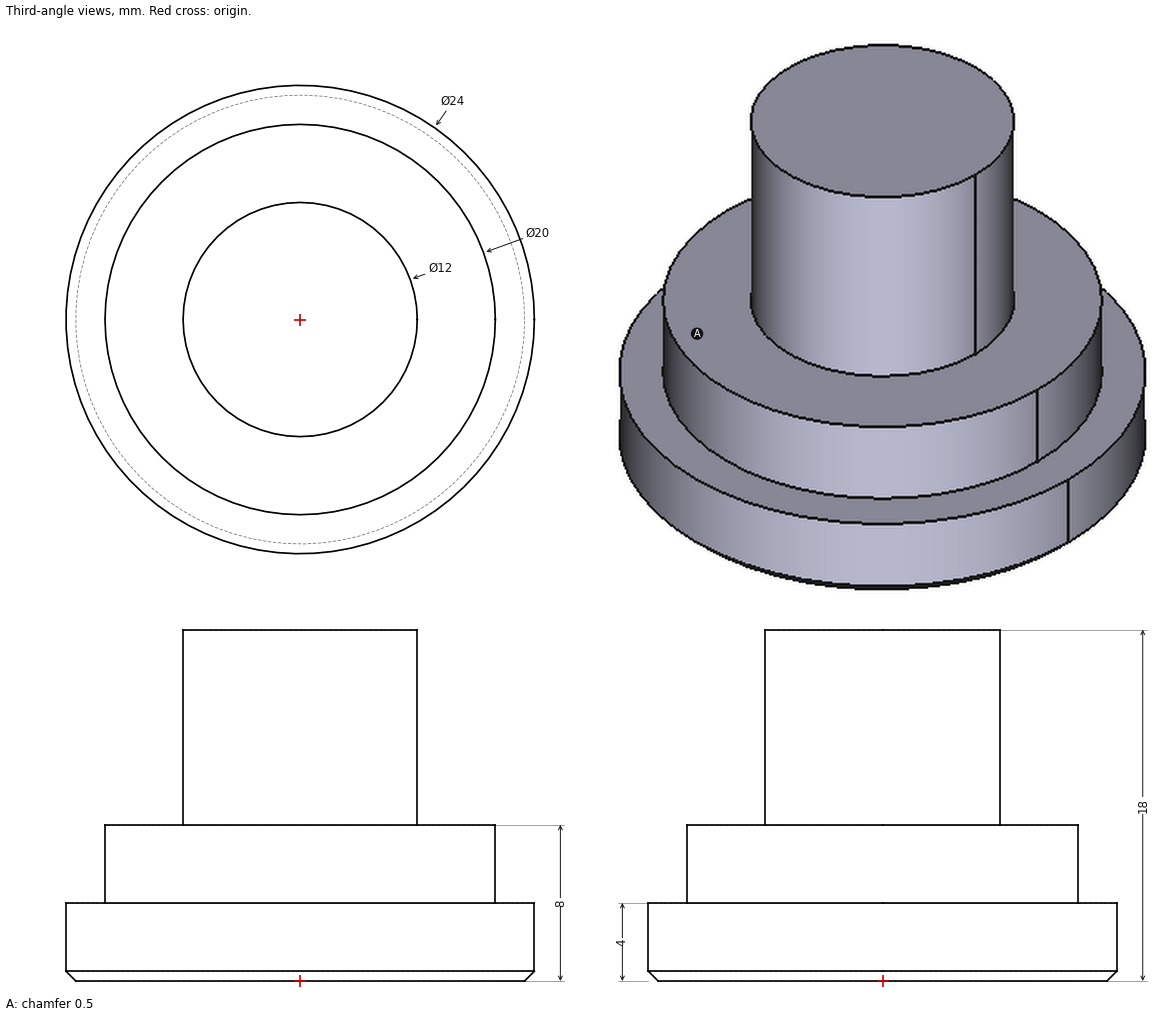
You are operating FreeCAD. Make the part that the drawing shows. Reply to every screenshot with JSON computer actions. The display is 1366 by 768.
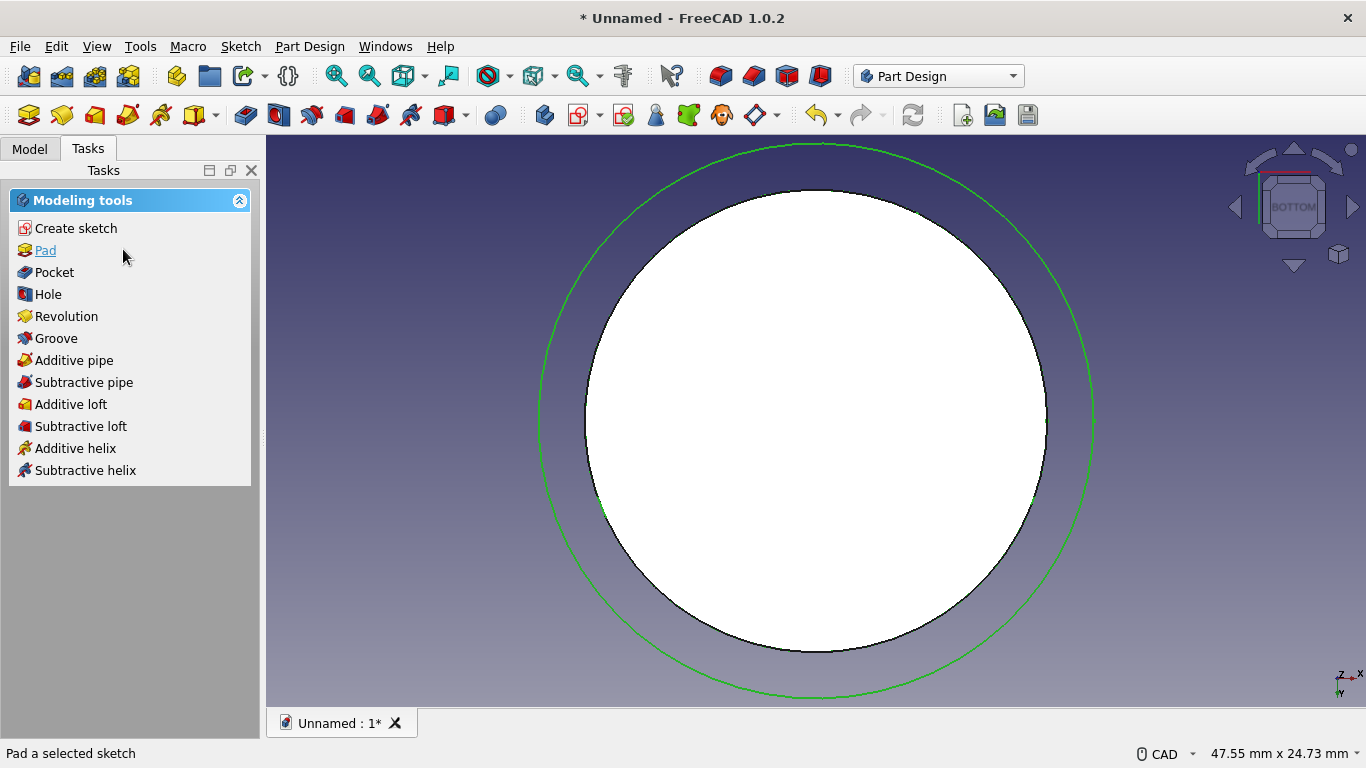
{"action": "left_click", "coordinate": [29, 116]}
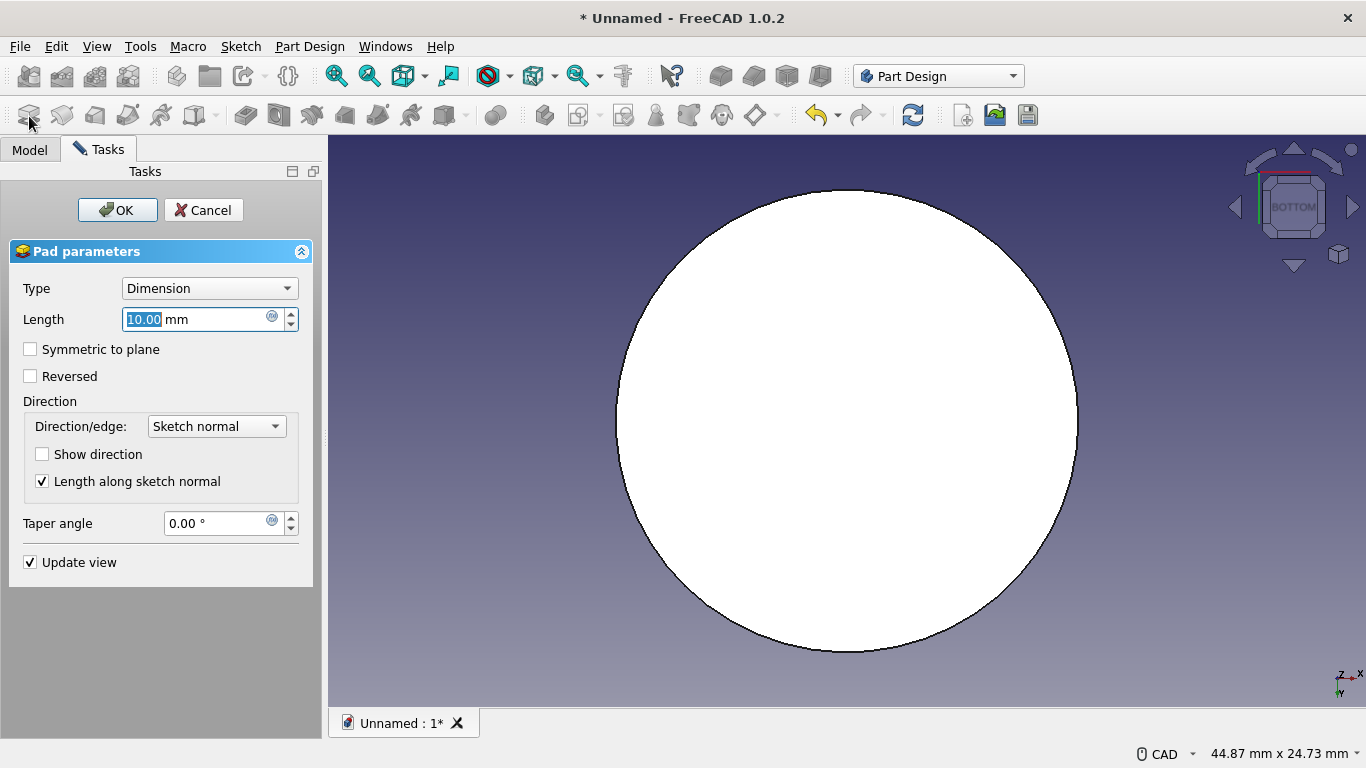
{"action": "type", "text": "4"}
{"action": "key", "text": "Tab"}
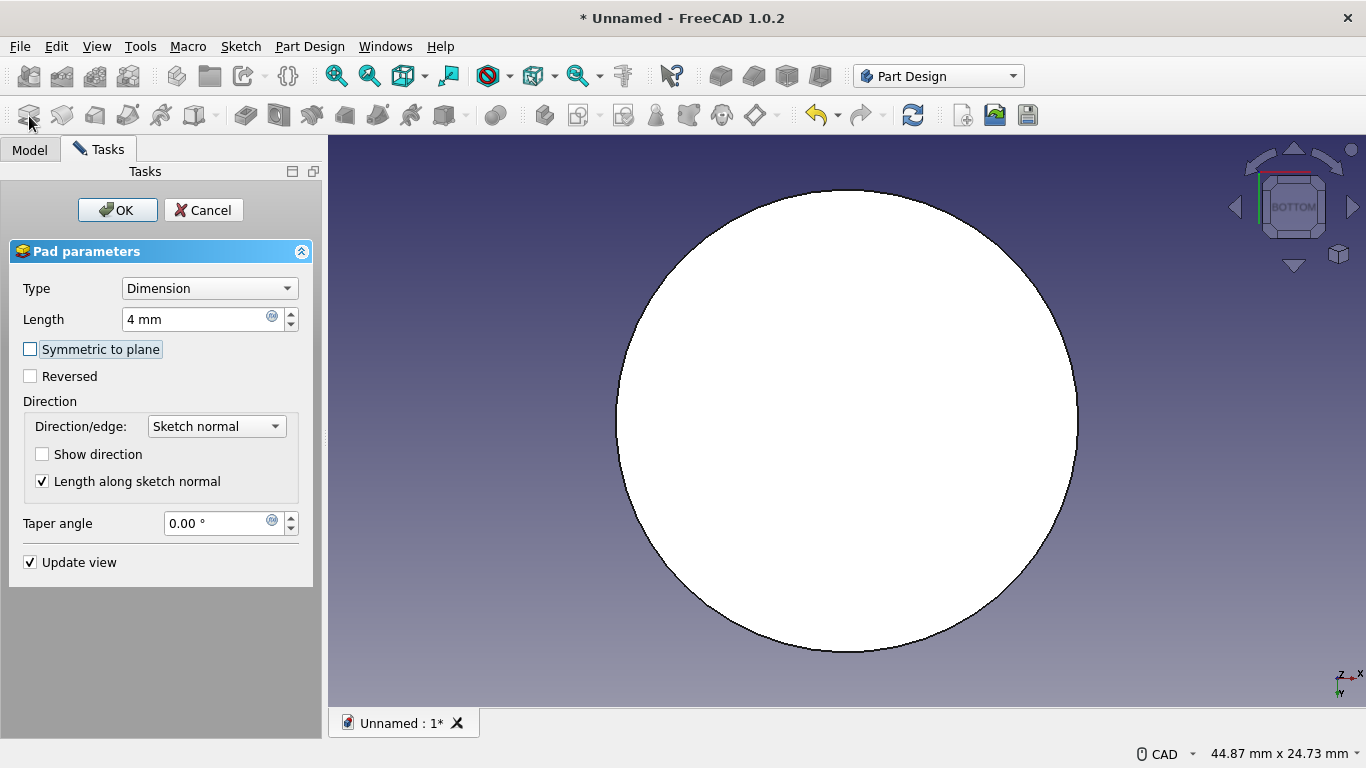
{"action": "left_click", "coordinate": [31, 376]}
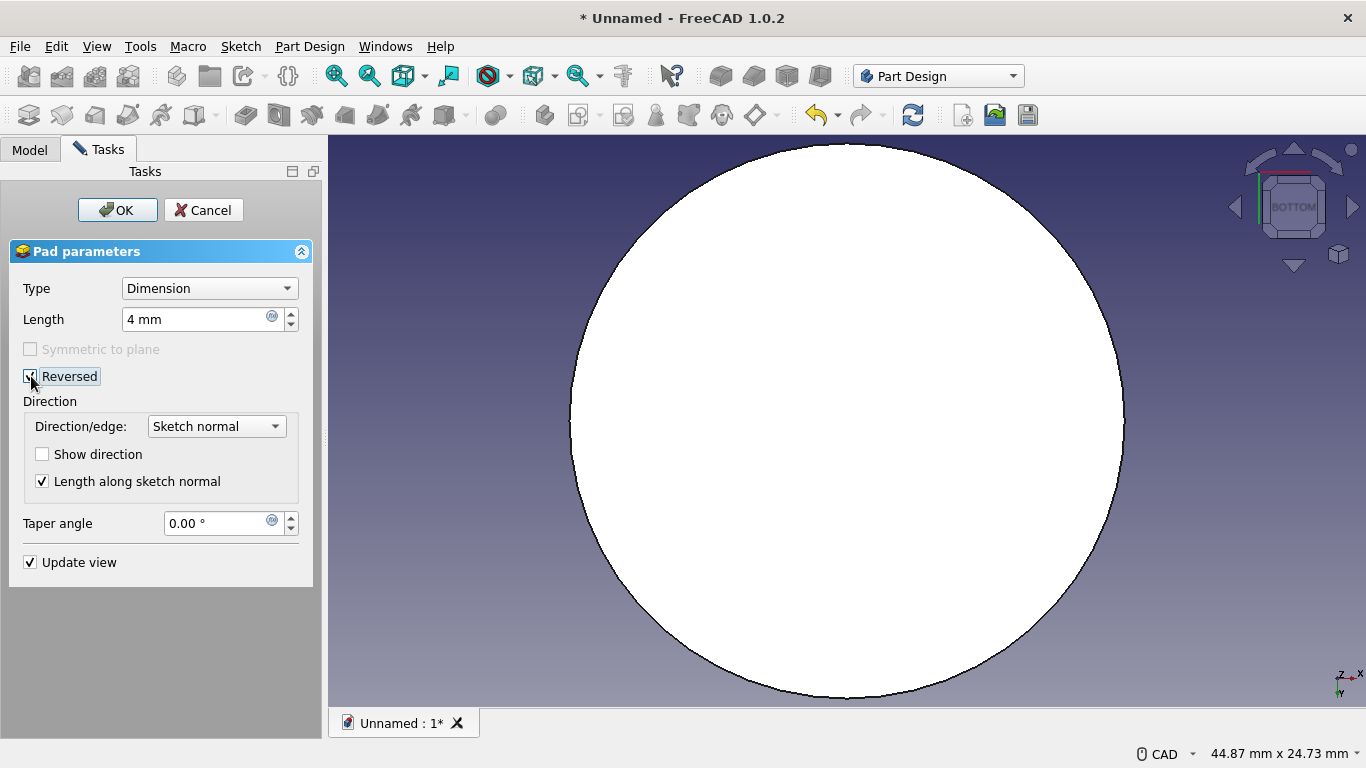
{"action": "left_click", "coordinate": [118, 210]}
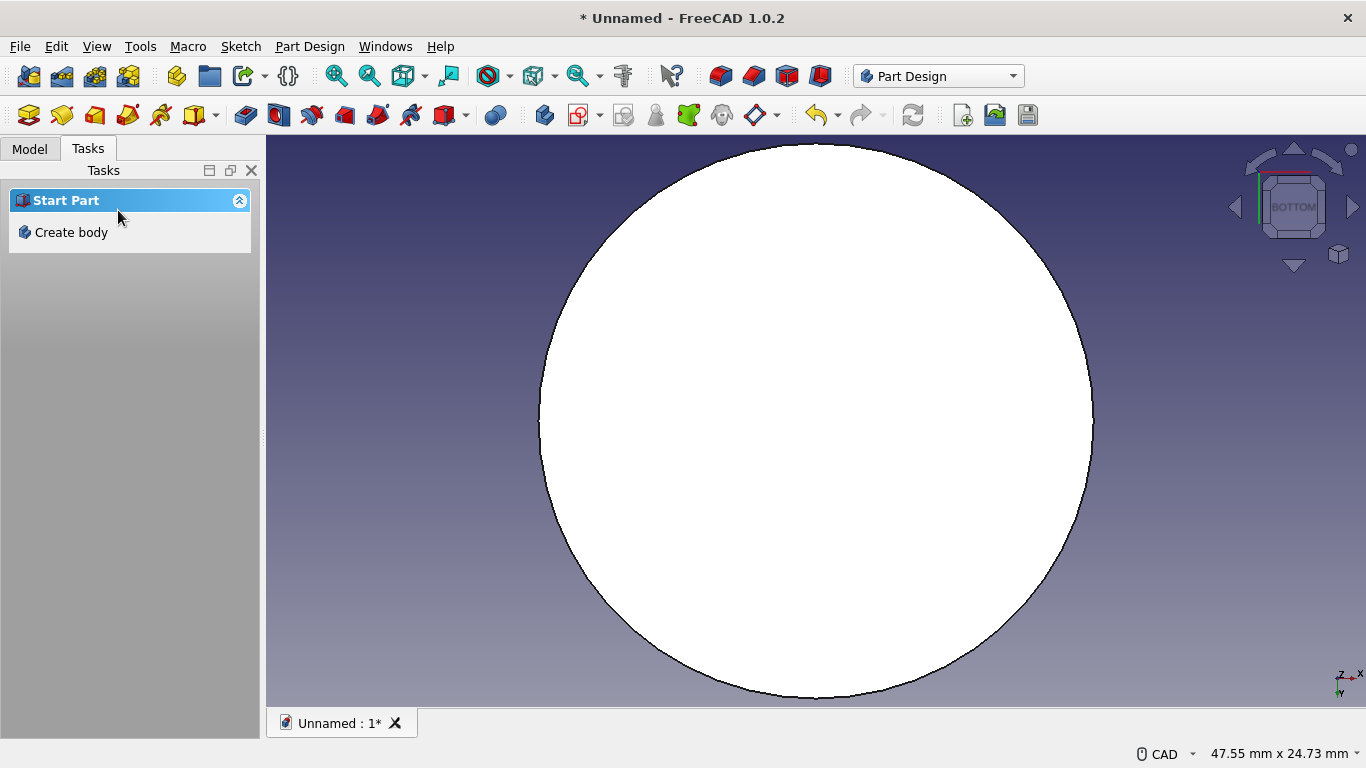
{"action": "left_click", "coordinate": [538, 420]}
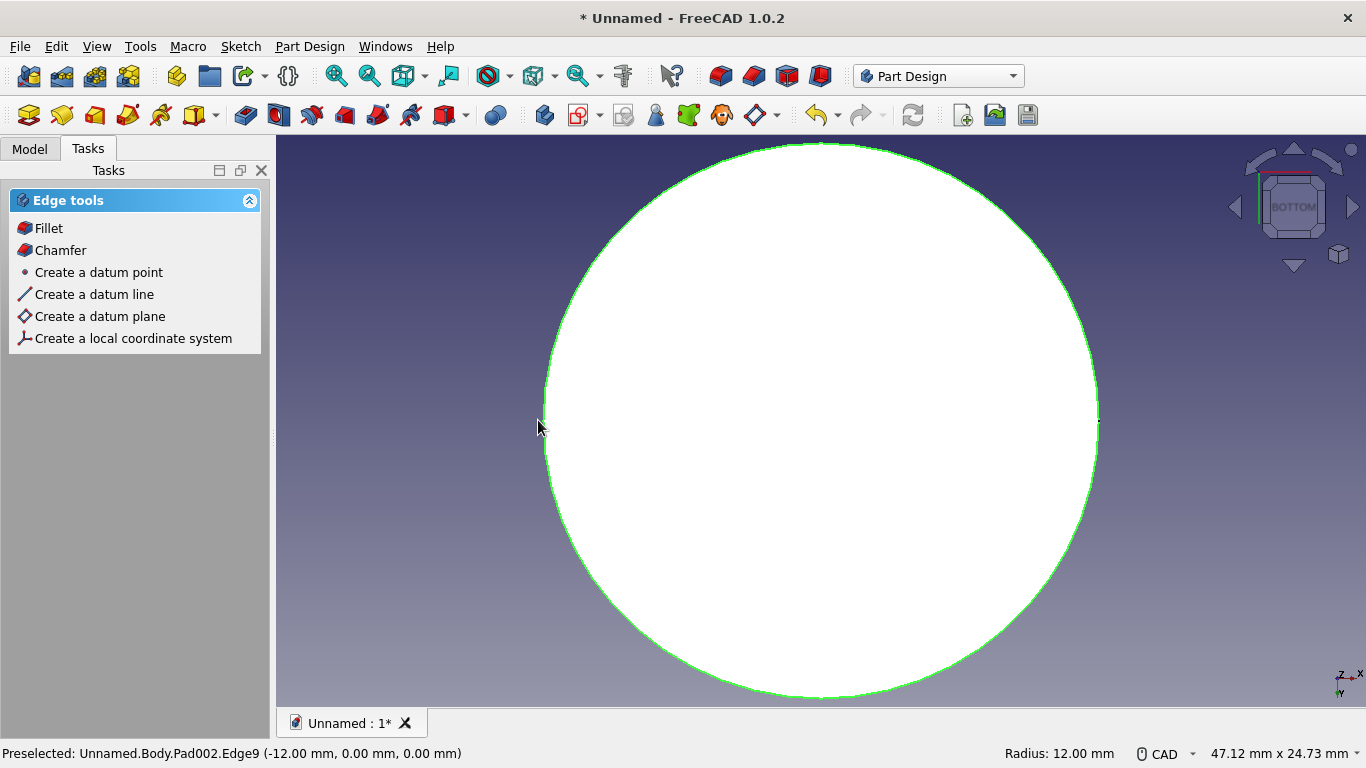
{"action": "left_click", "coordinate": [754, 76]}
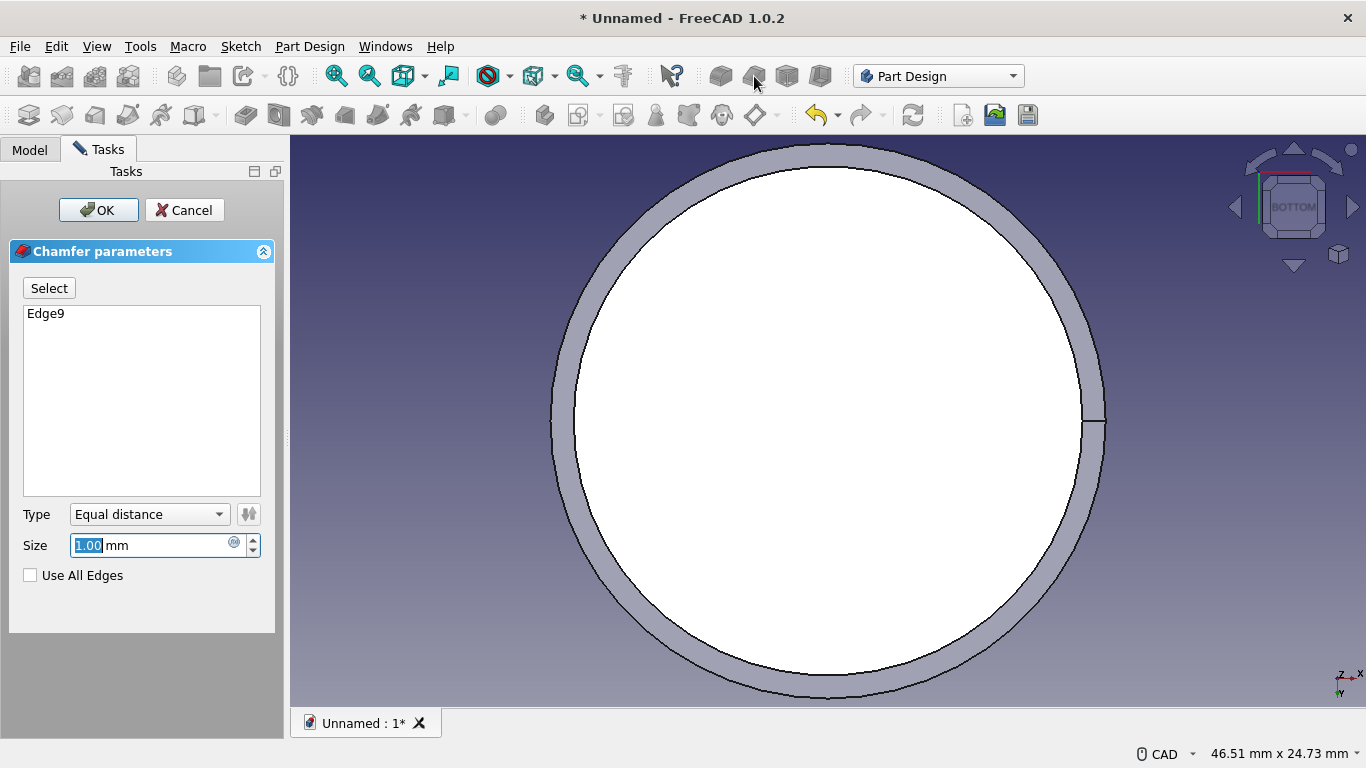
{"action": "type", "text": "0.5"}
{"action": "key", "text": "Tab"}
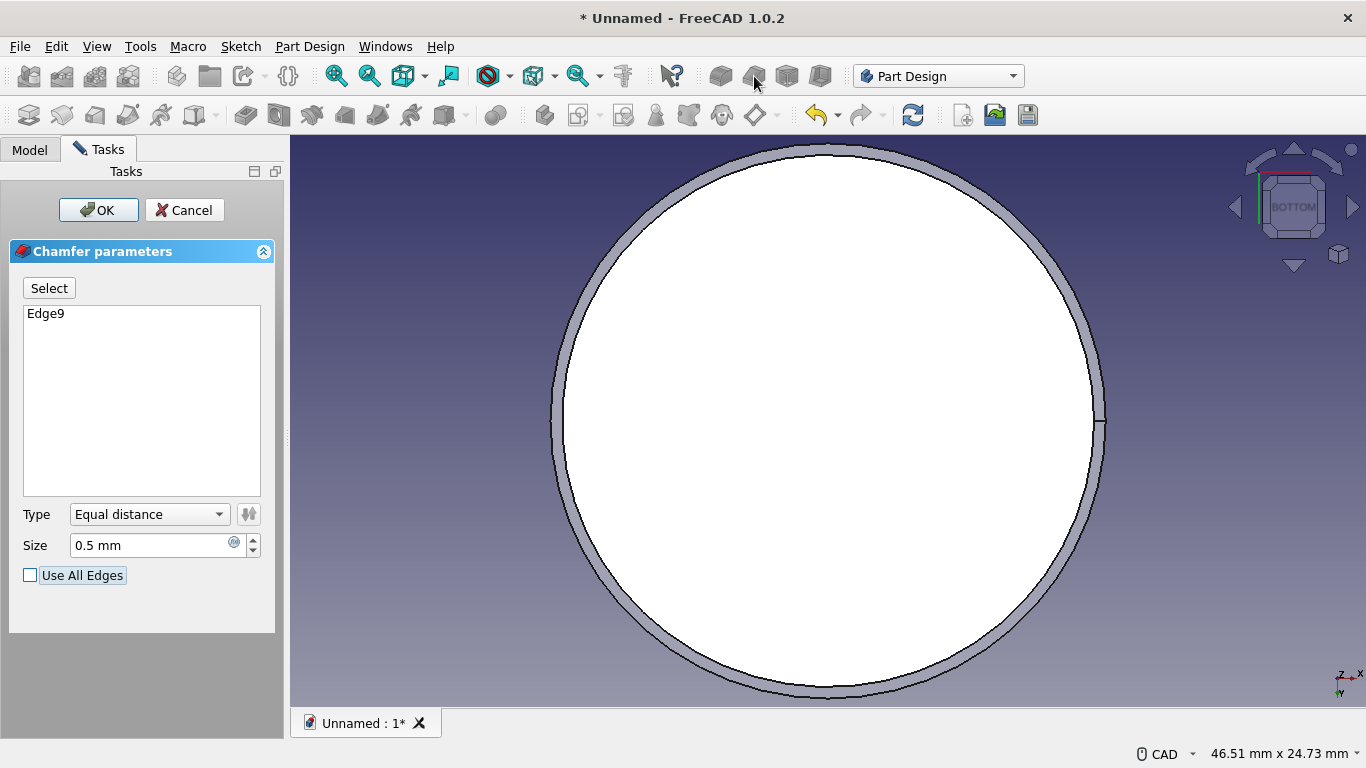
{"action": "left_click", "coordinate": [99, 210]}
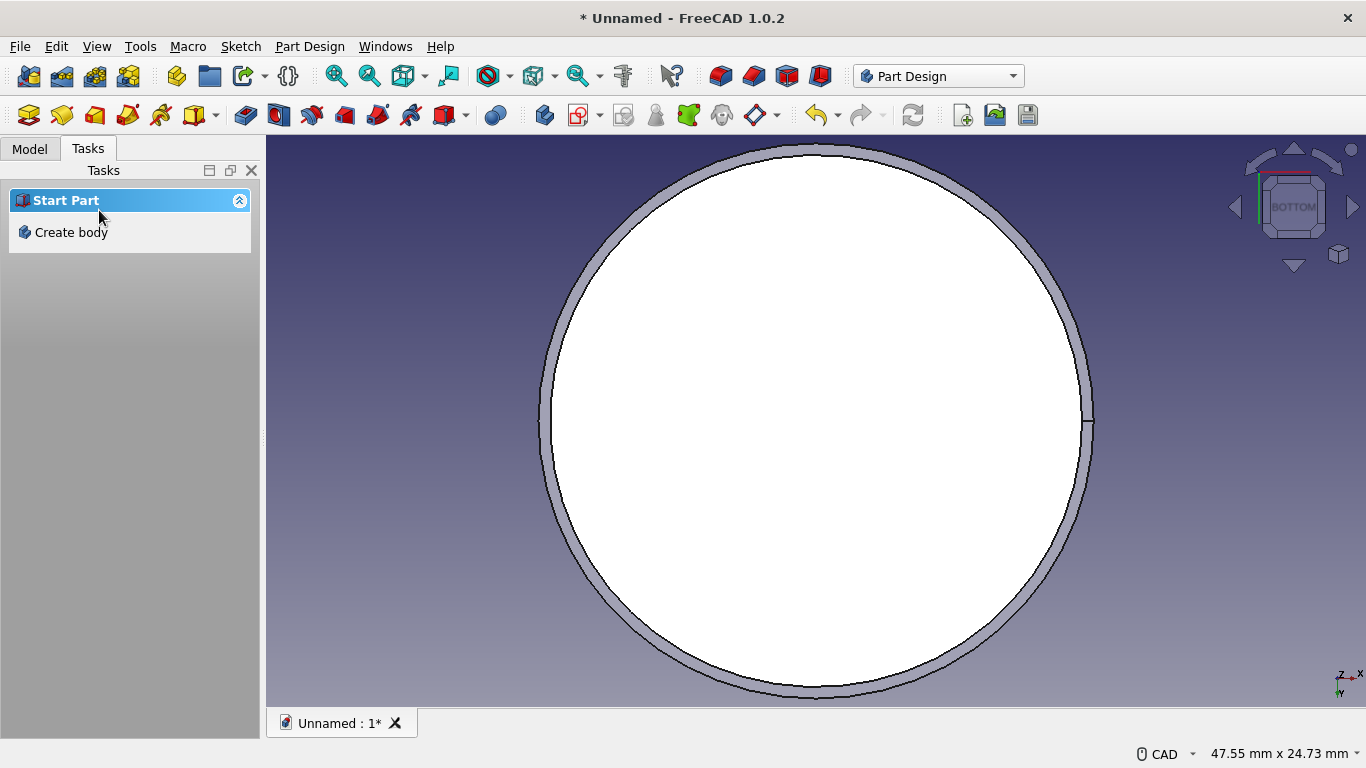
{"action": "key", "text": "0"}